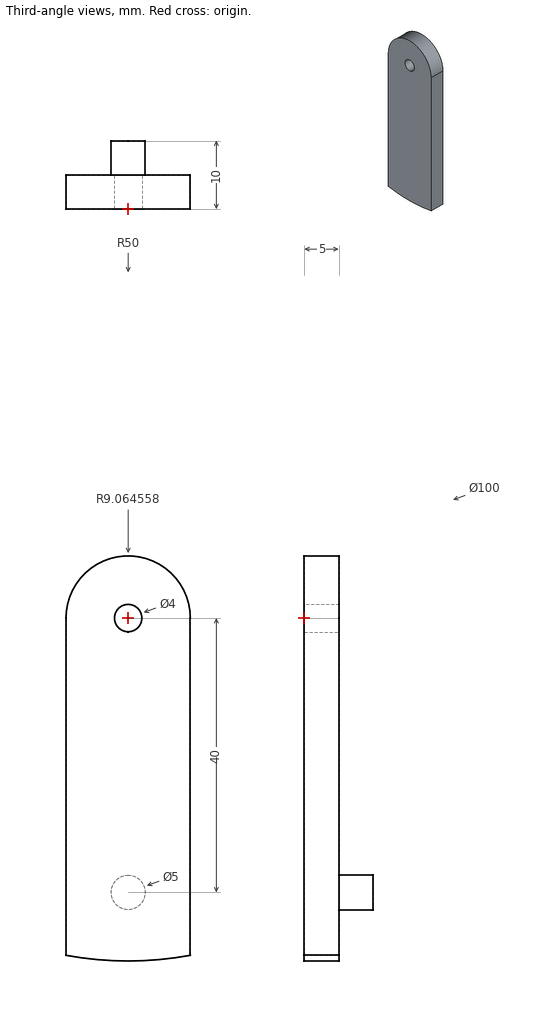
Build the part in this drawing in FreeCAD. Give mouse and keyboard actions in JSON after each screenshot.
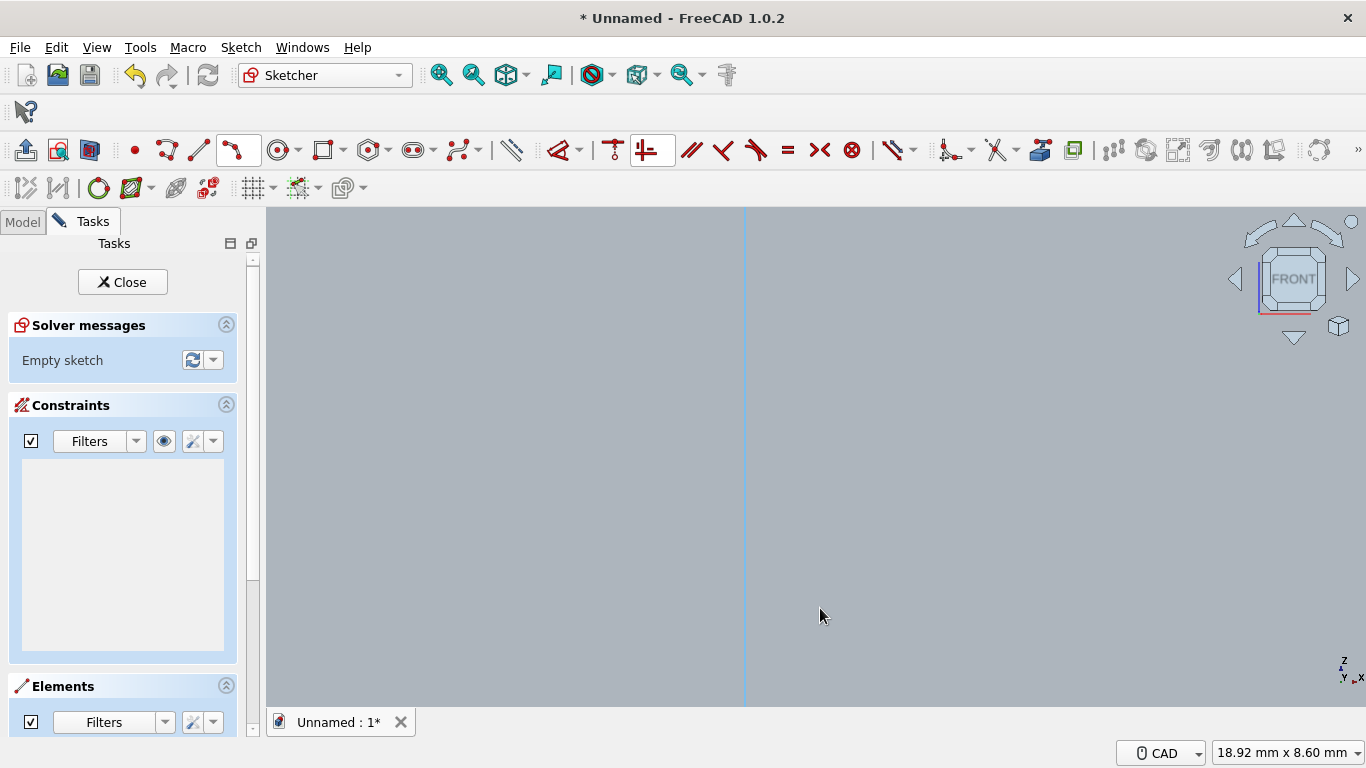
{"action": "key", "text": "g c"}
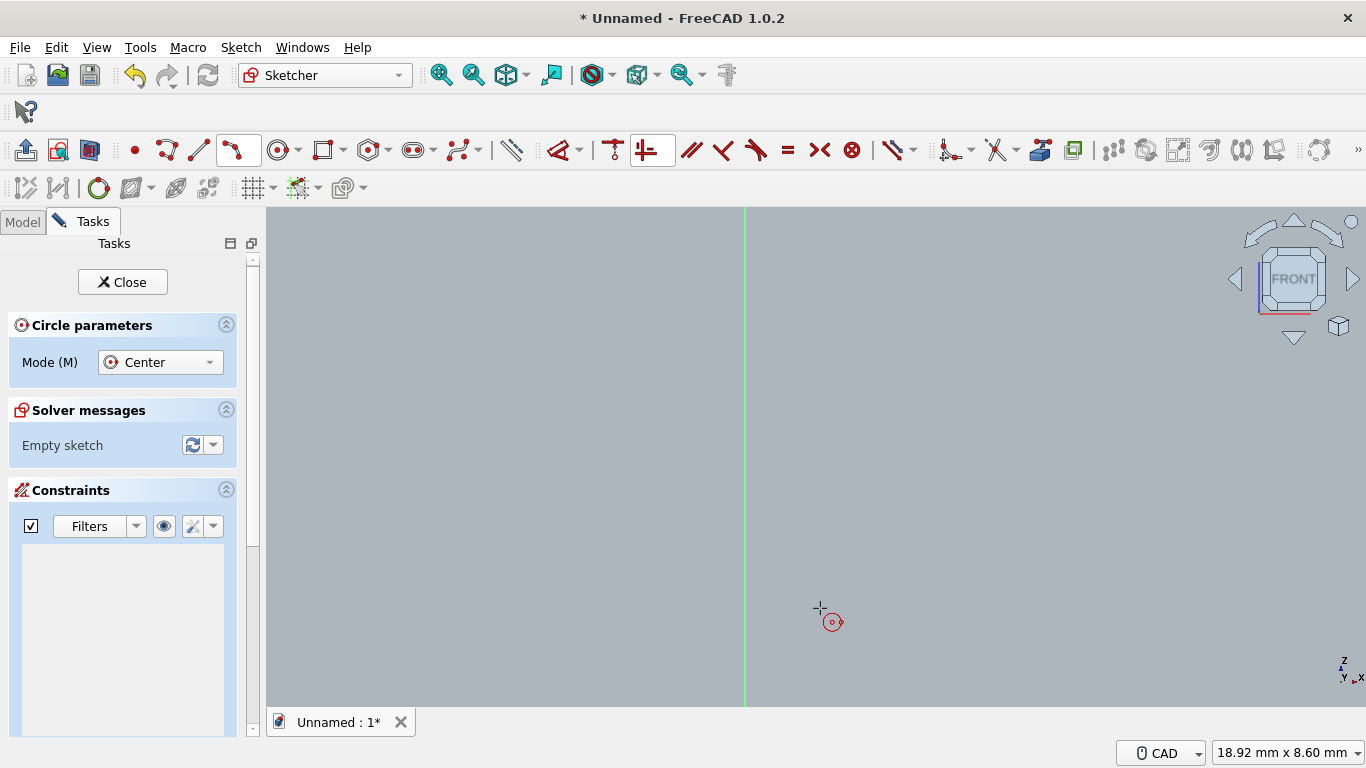
{"action": "left_click", "coordinate": [745, 438]}
{"action": "left_click", "coordinate": [847, 335]}
{"action": "key", "text": "Escape"}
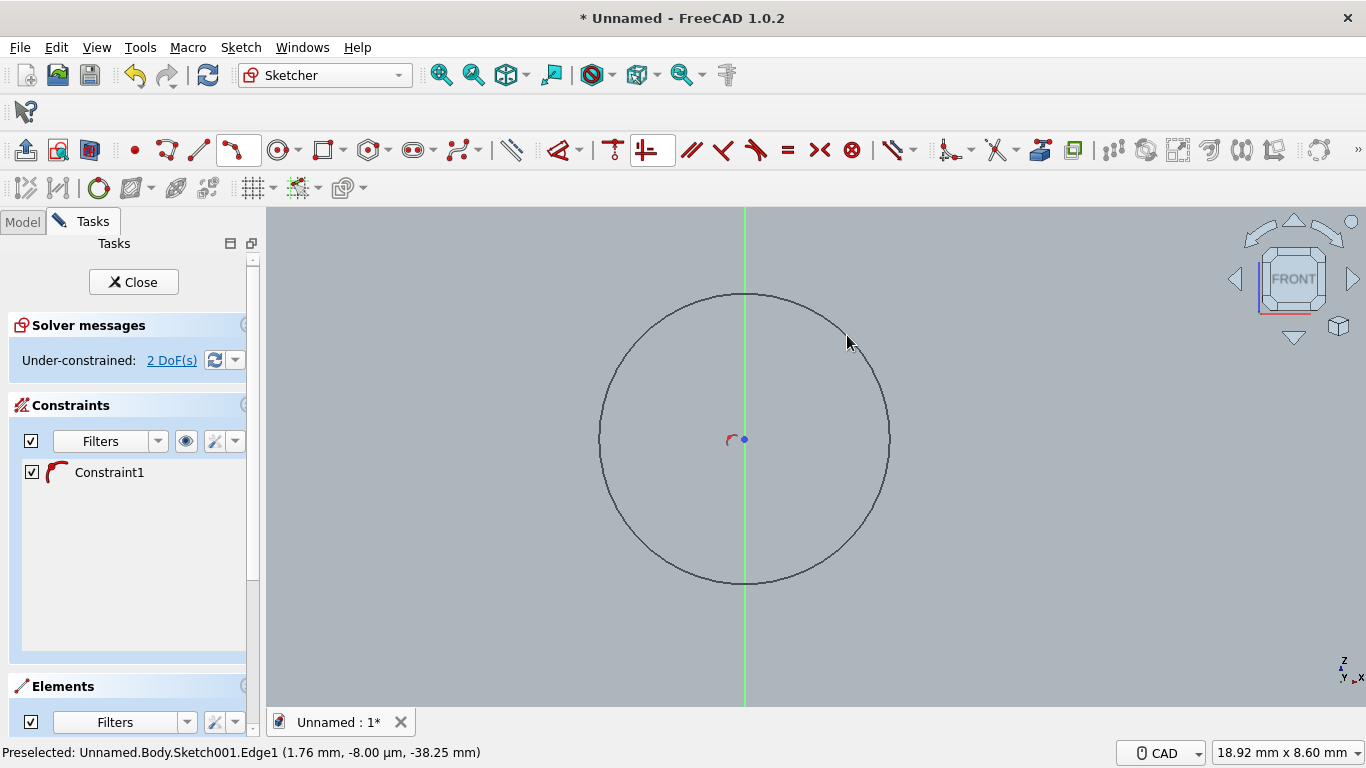
{"action": "left_click", "coordinate": [847, 336]}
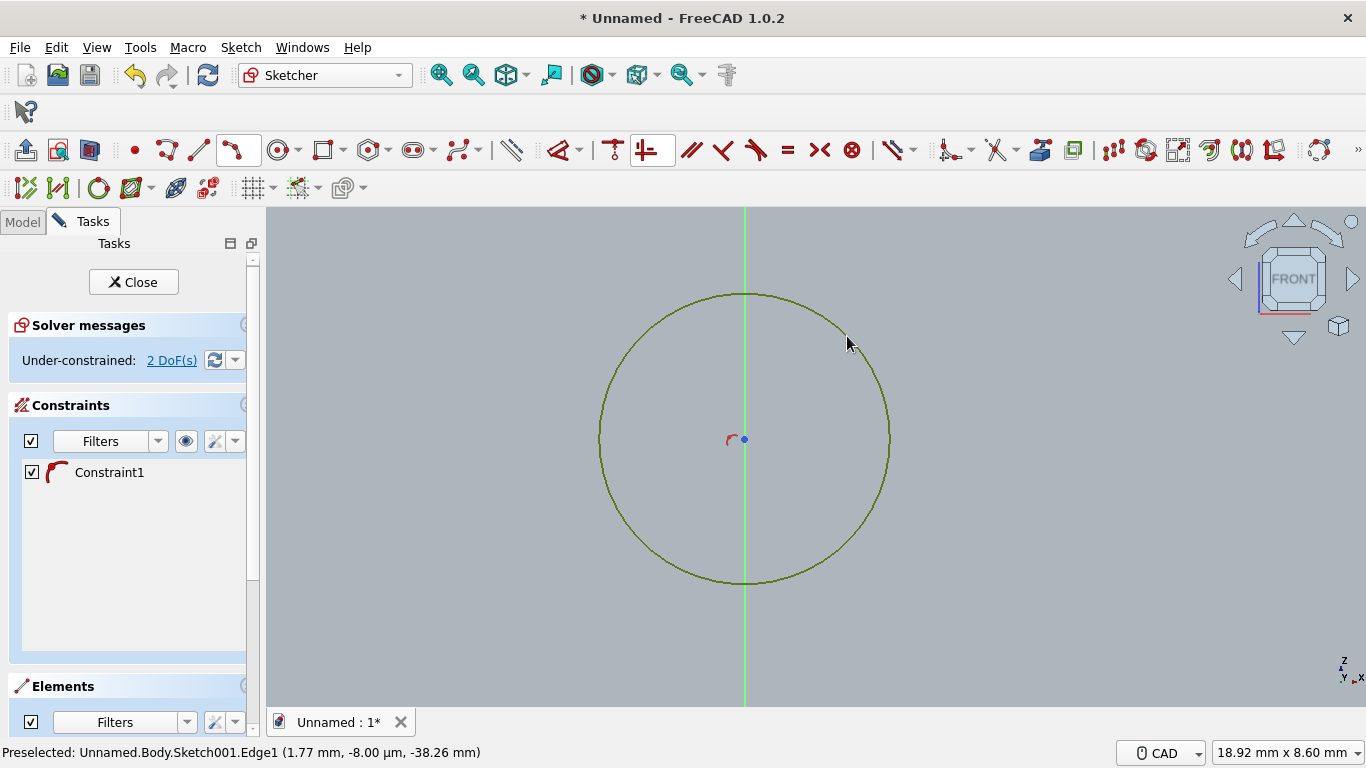
{"action": "key", "text": "k o"}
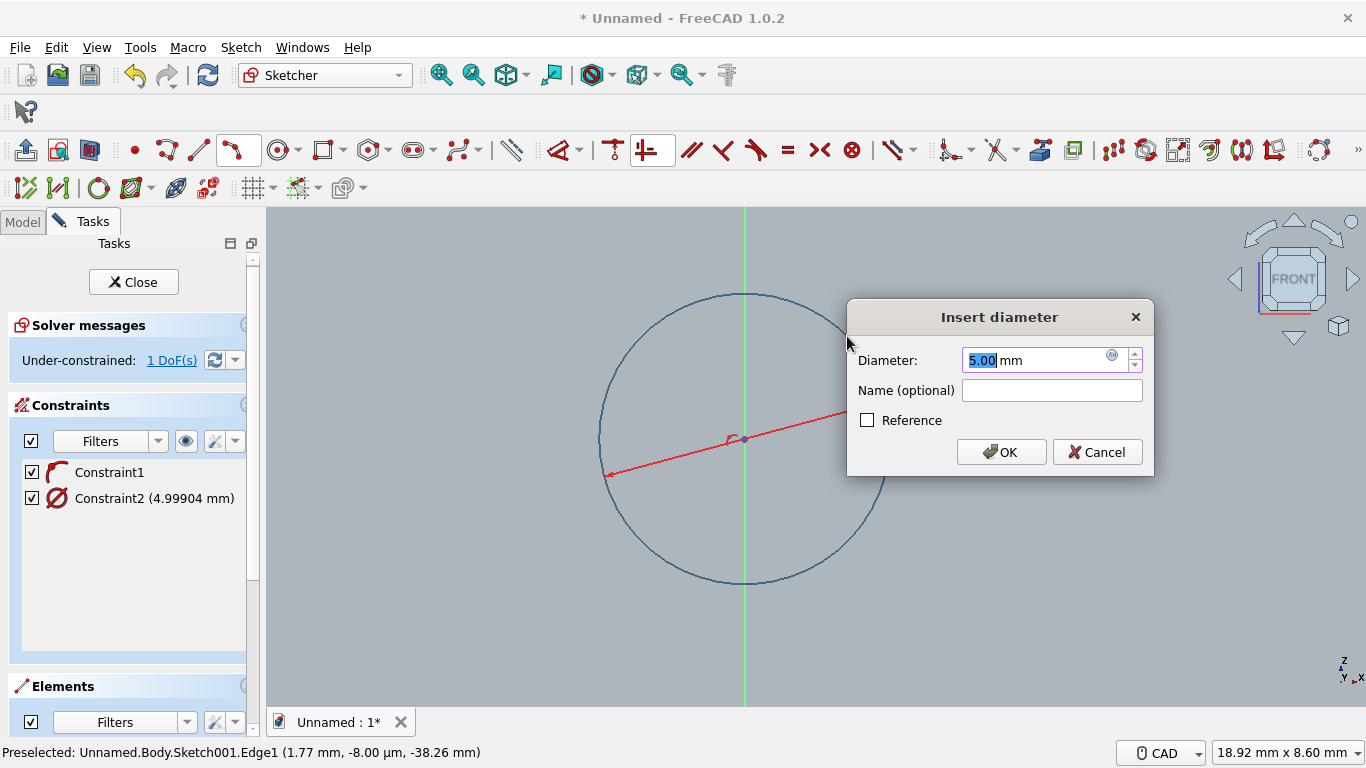
{"action": "type", "text": "5"}
{"action": "key", "text": "Return"}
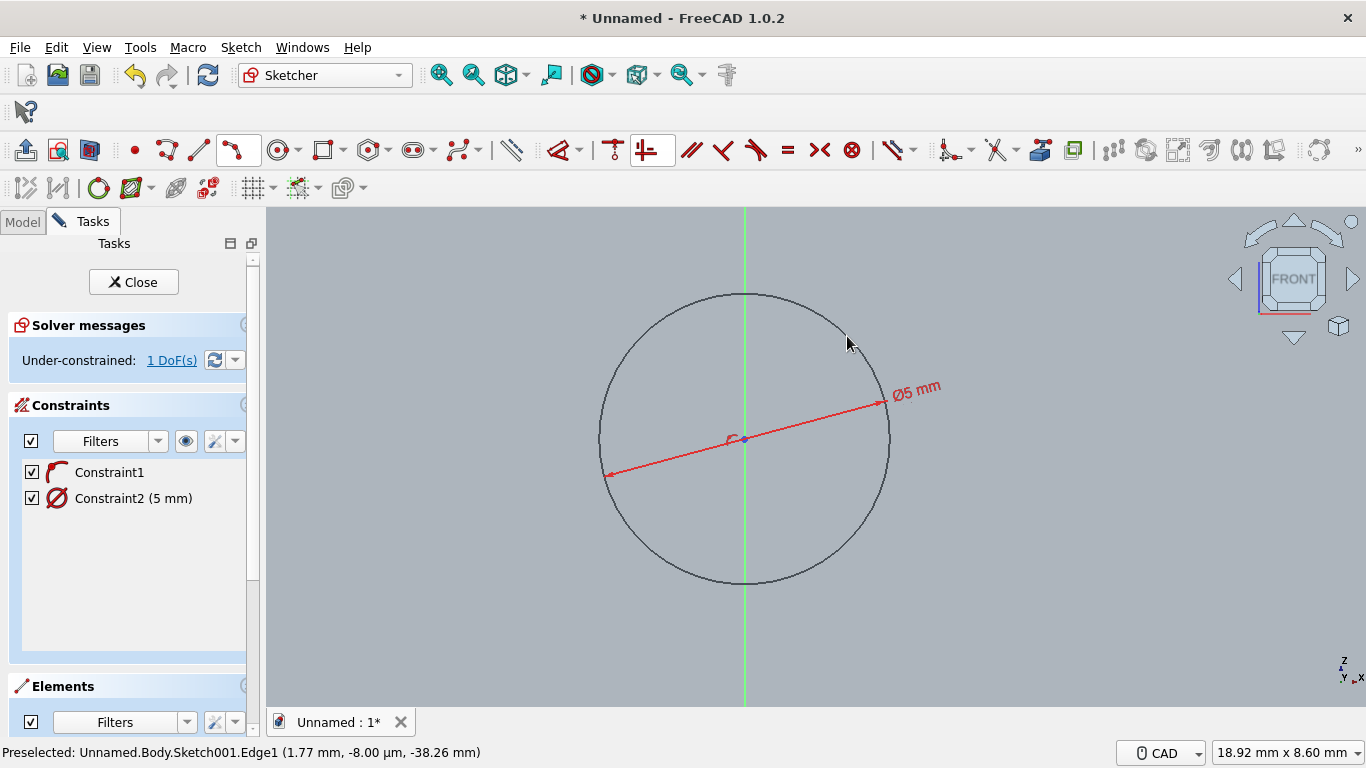
{"action": "left_click", "coordinate": [745, 439]}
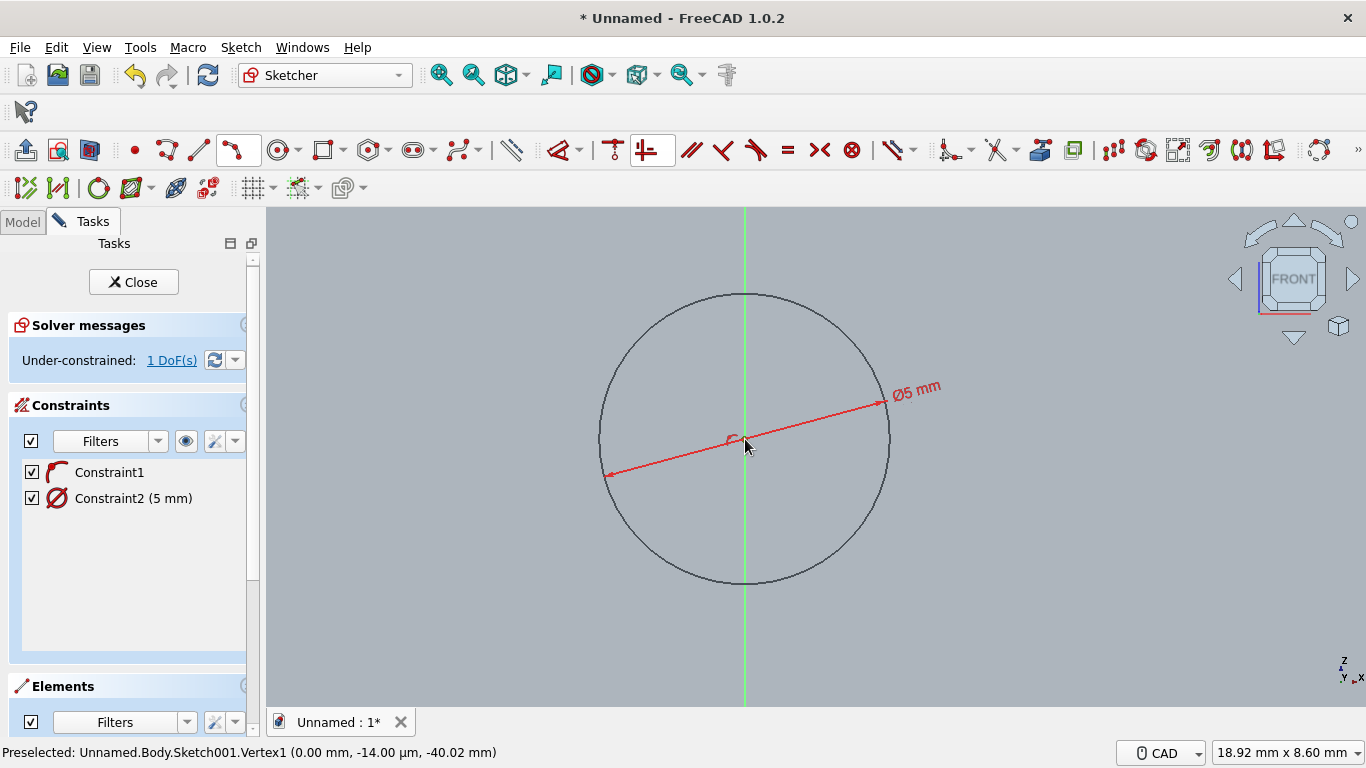
{"action": "key", "text": "i"}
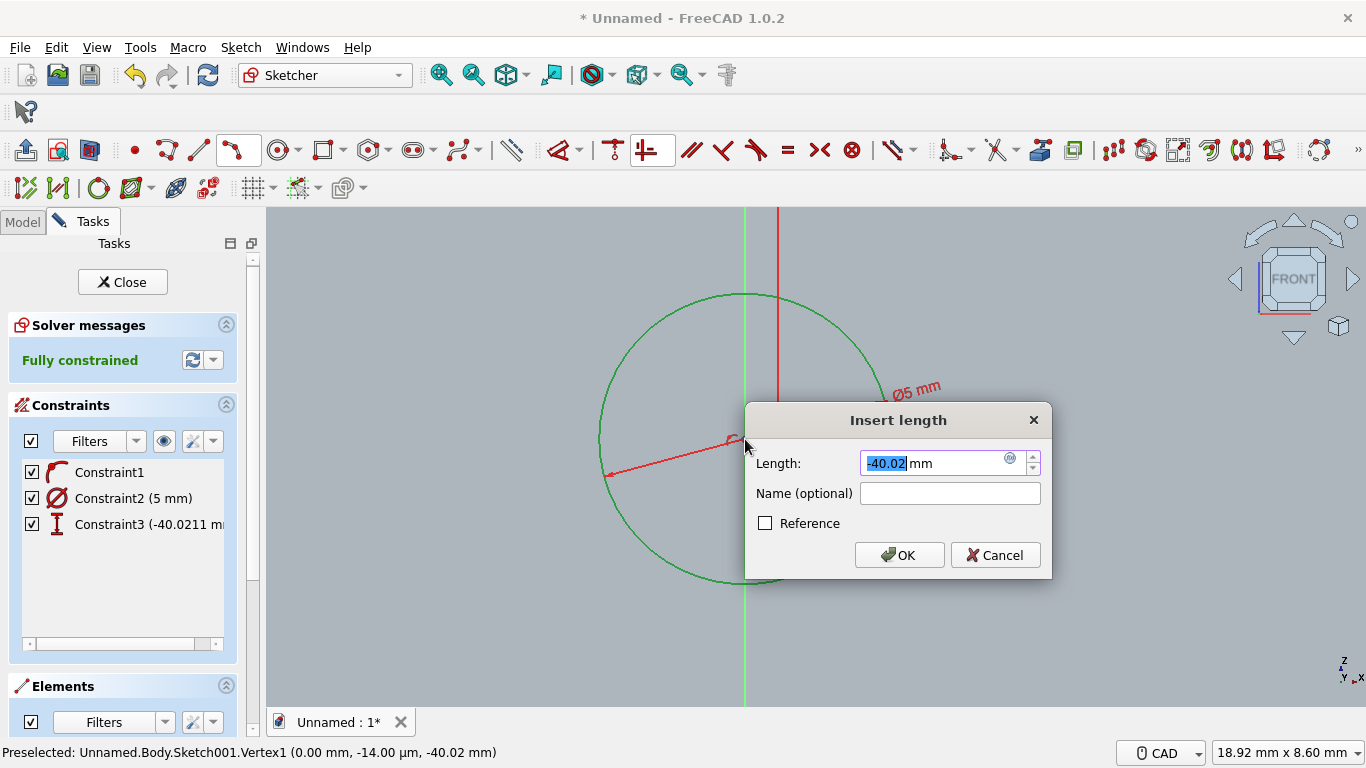
{"action": "type", "text": "-40"}
{"action": "key", "text": "Return"}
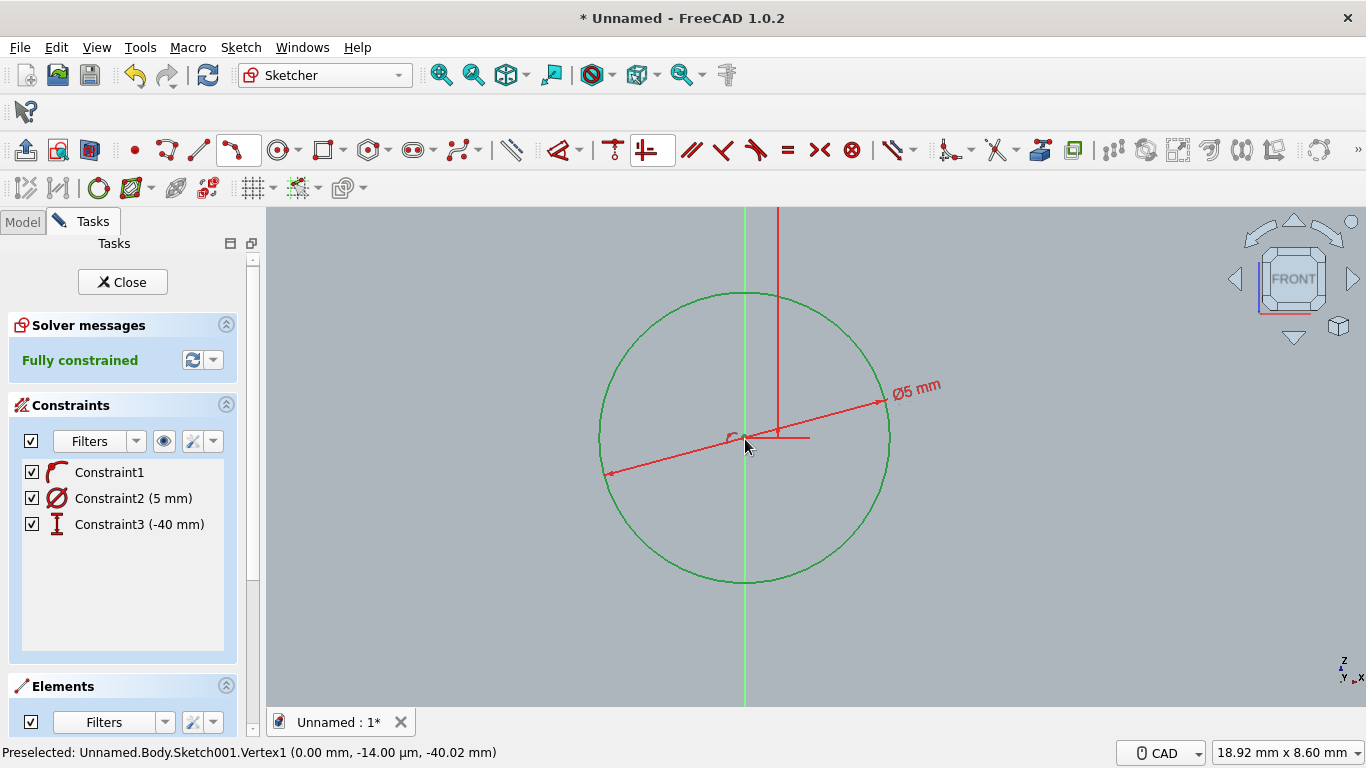
{"action": "left_click", "coordinate": [123, 282]}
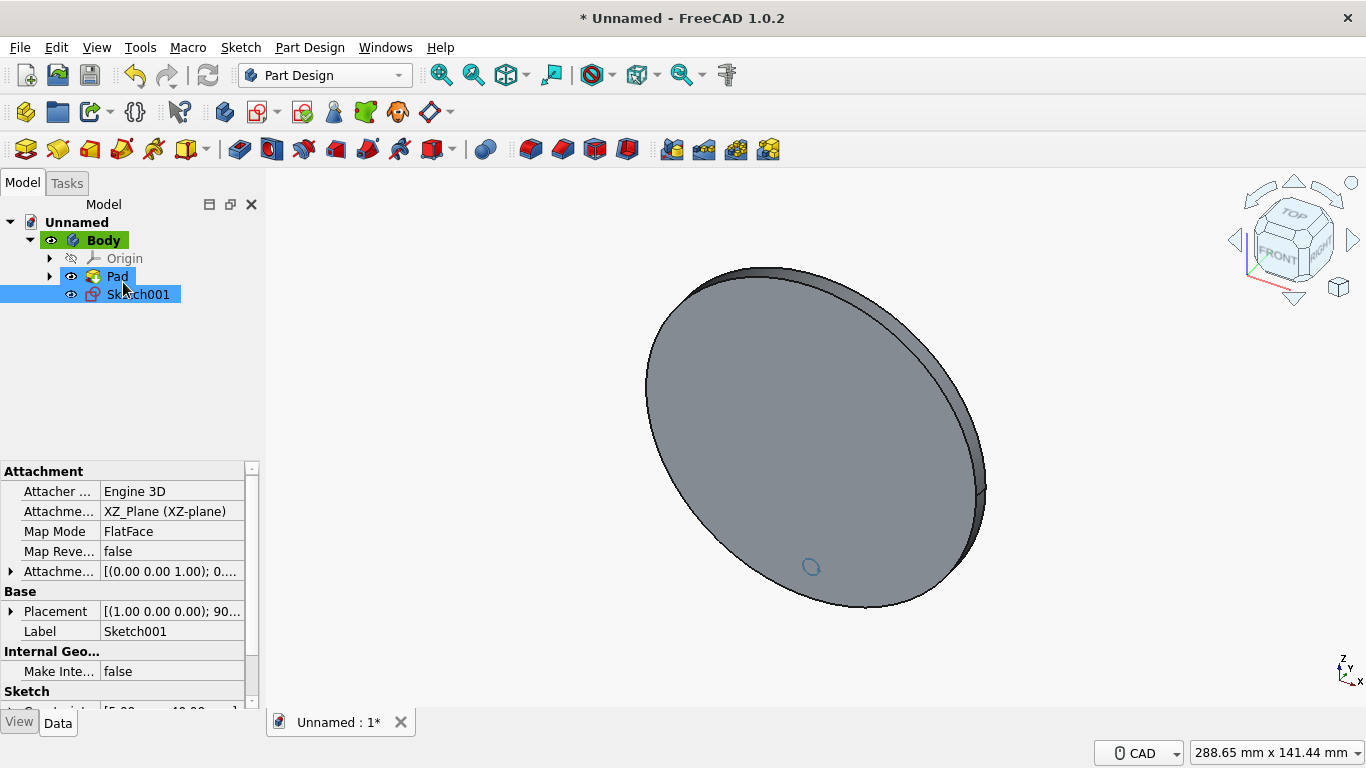
{"action": "left_click", "coordinate": [26, 150]}